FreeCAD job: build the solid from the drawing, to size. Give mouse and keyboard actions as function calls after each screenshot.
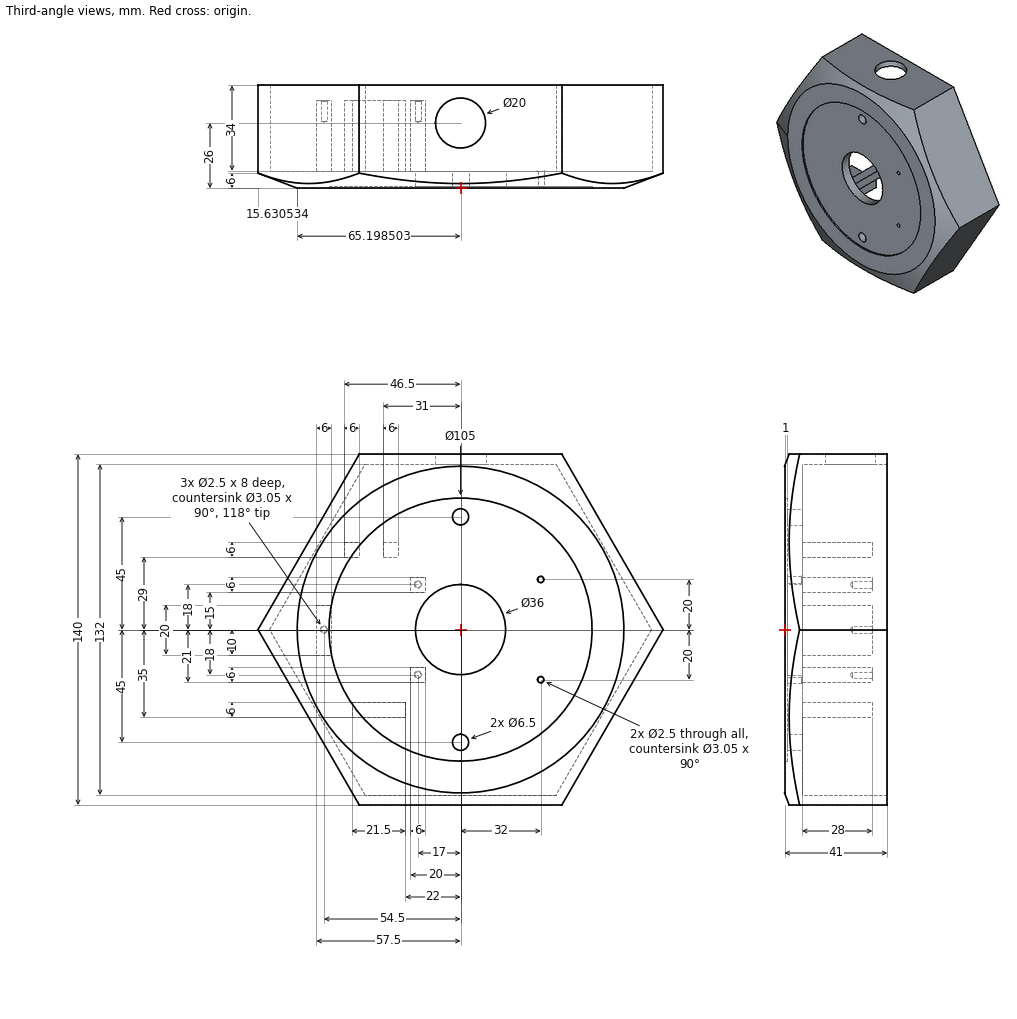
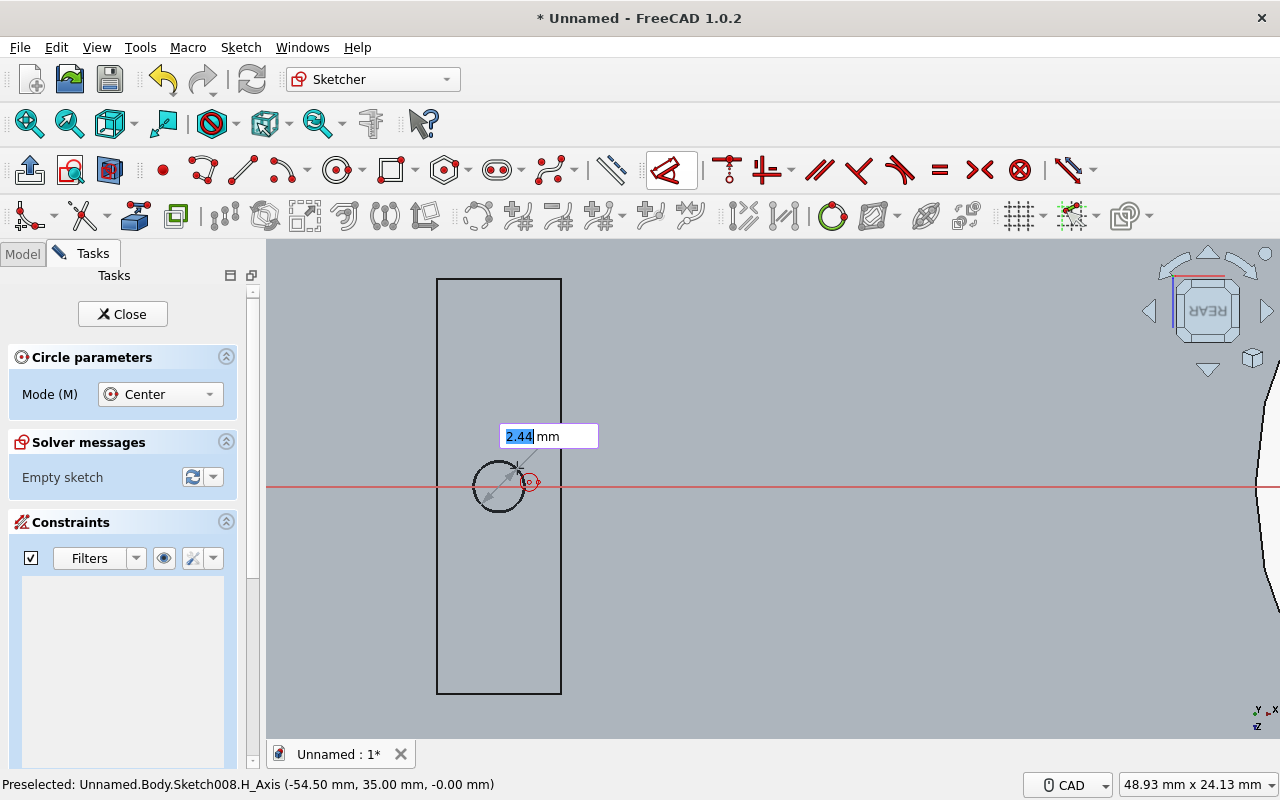
text(2.5)
key(Return)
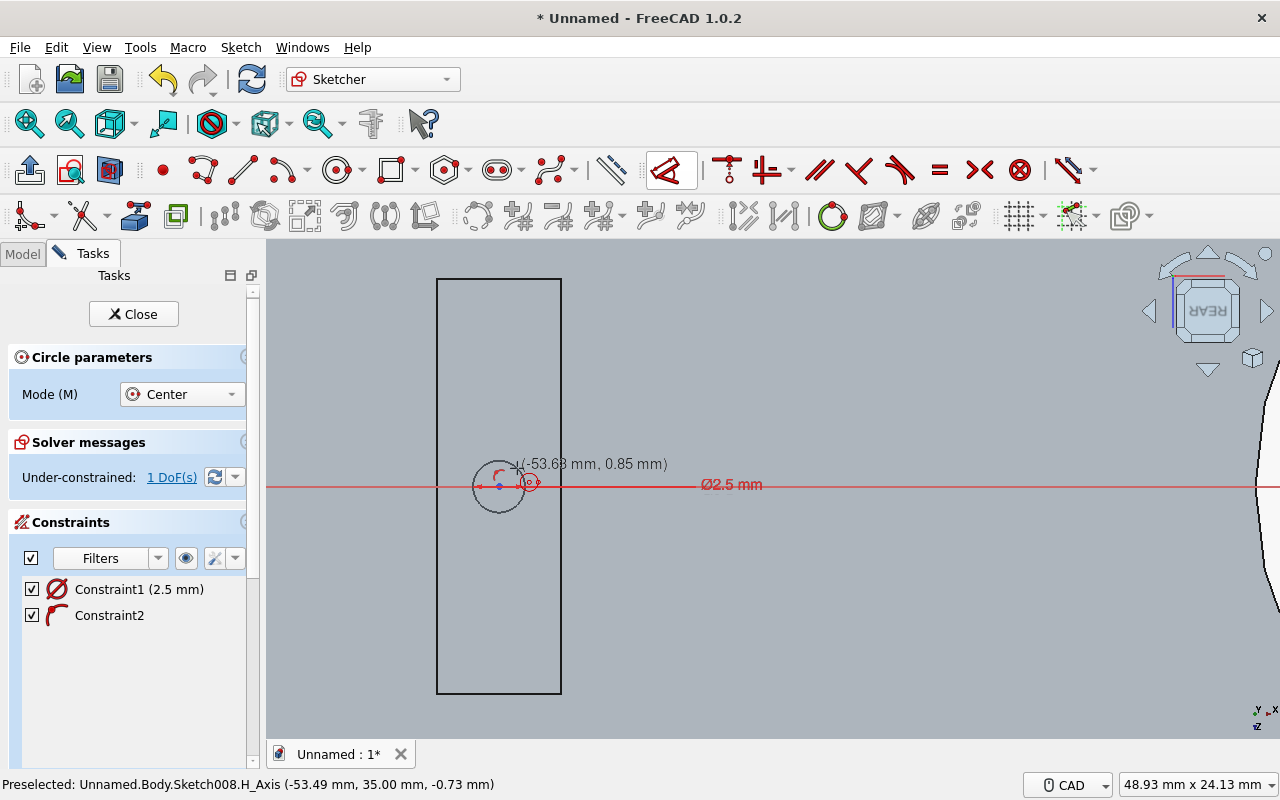
scroll(503, 490, down, 5)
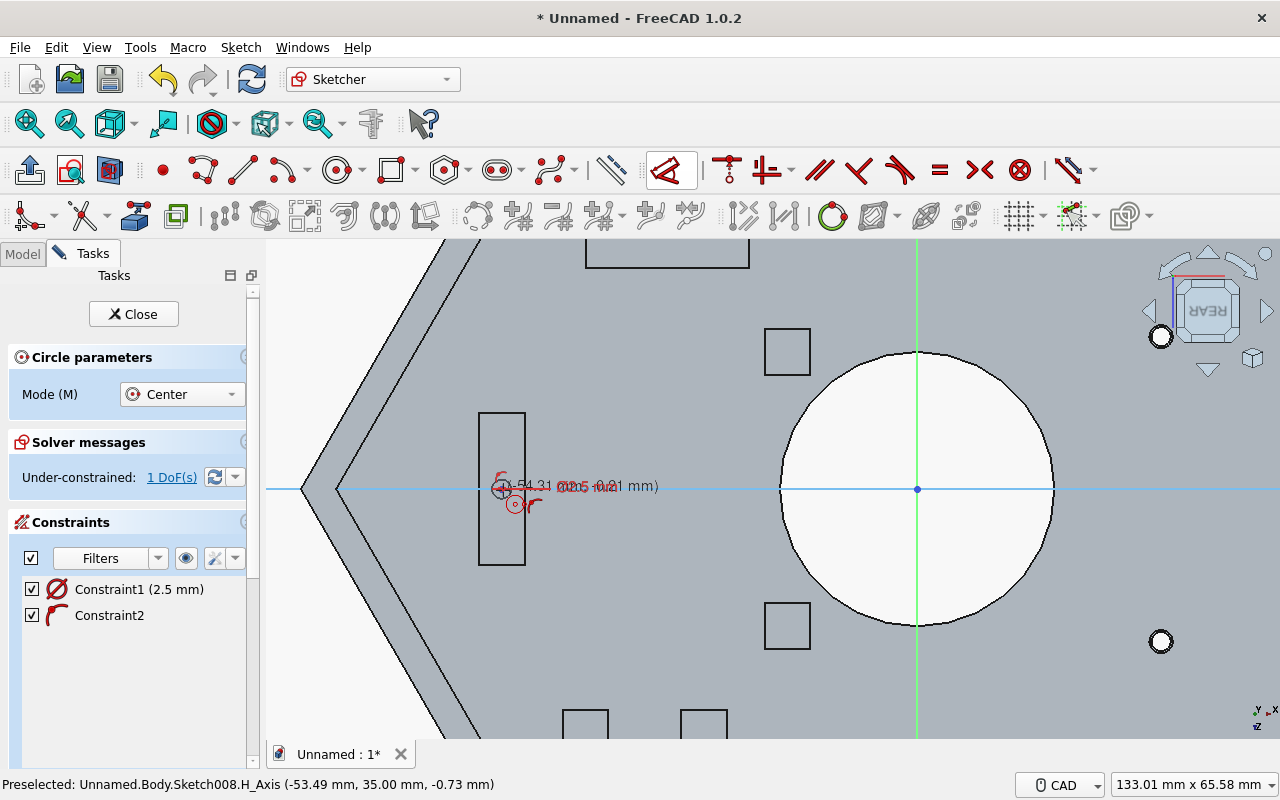
scroll(788, 352, up, 5)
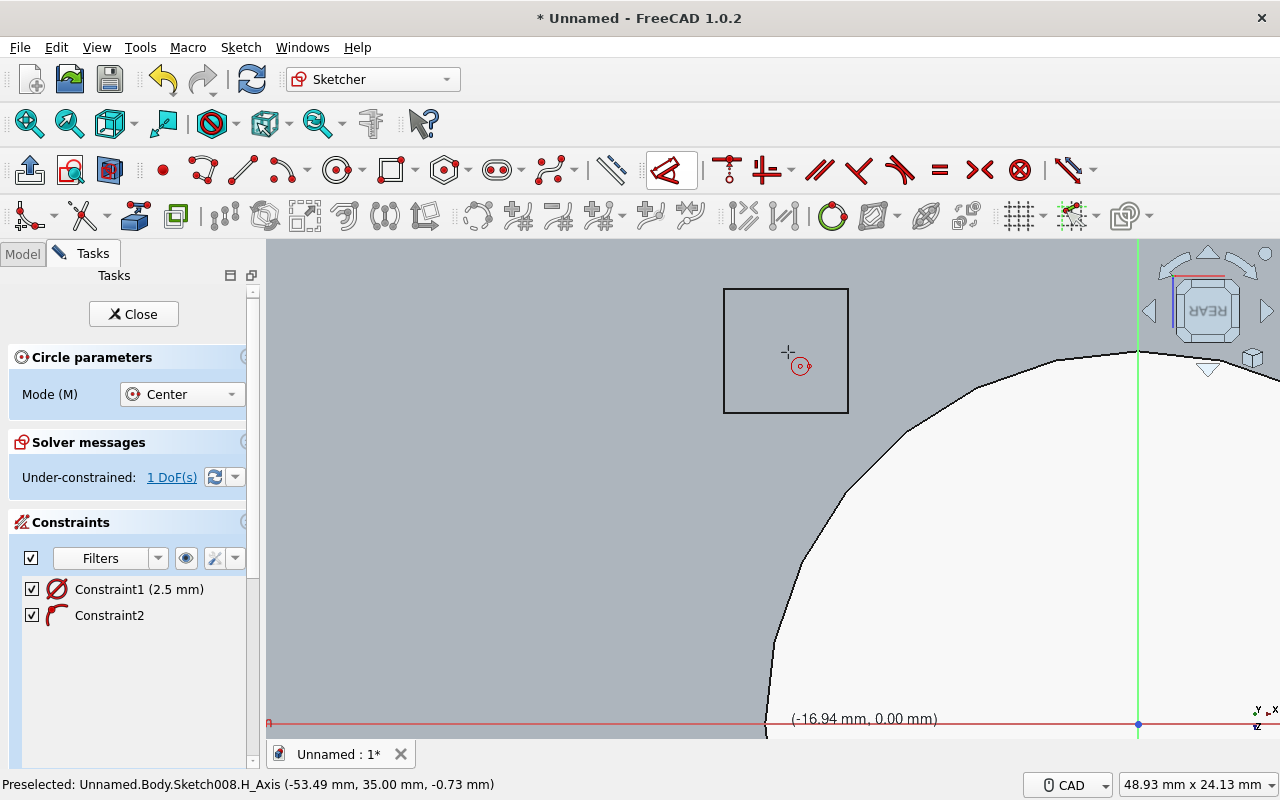
click(786, 351)
move(804, 333)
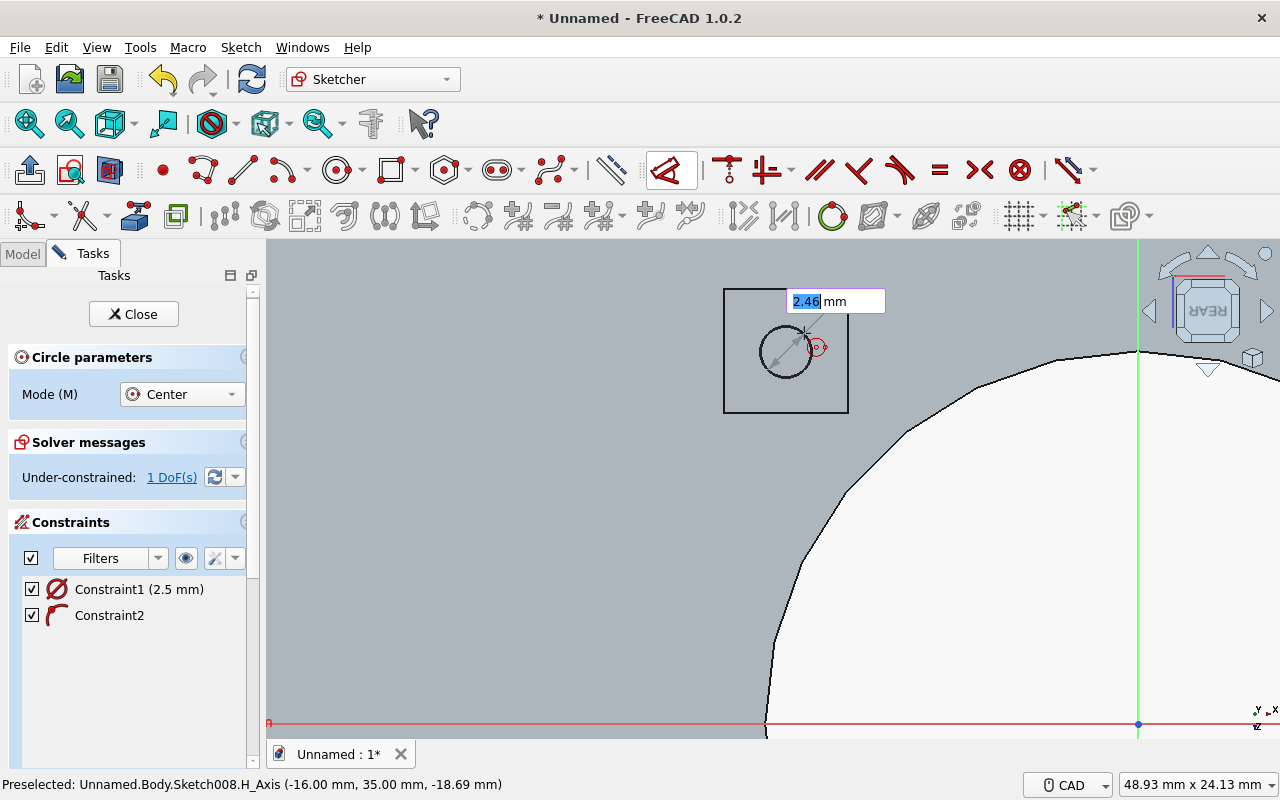
text(2.5)
key(Return)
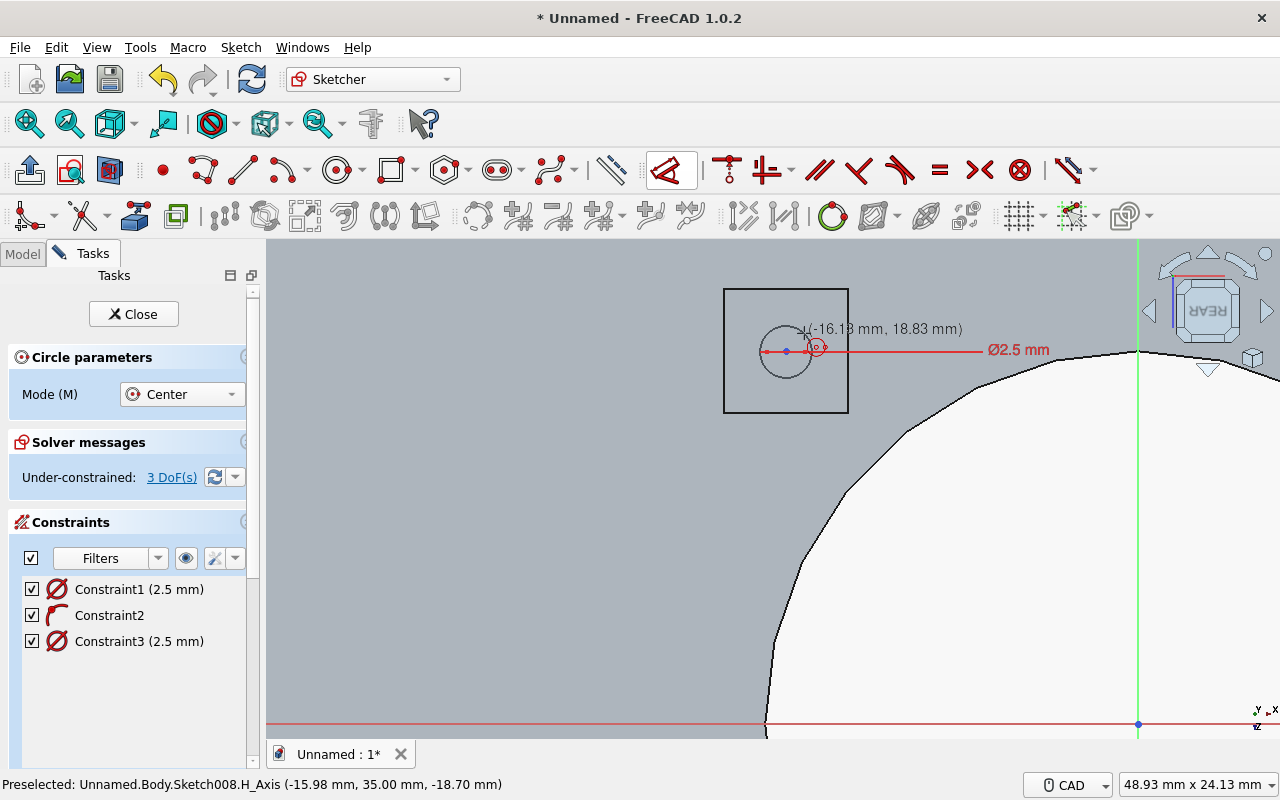
scroll(788, 352, down, 5)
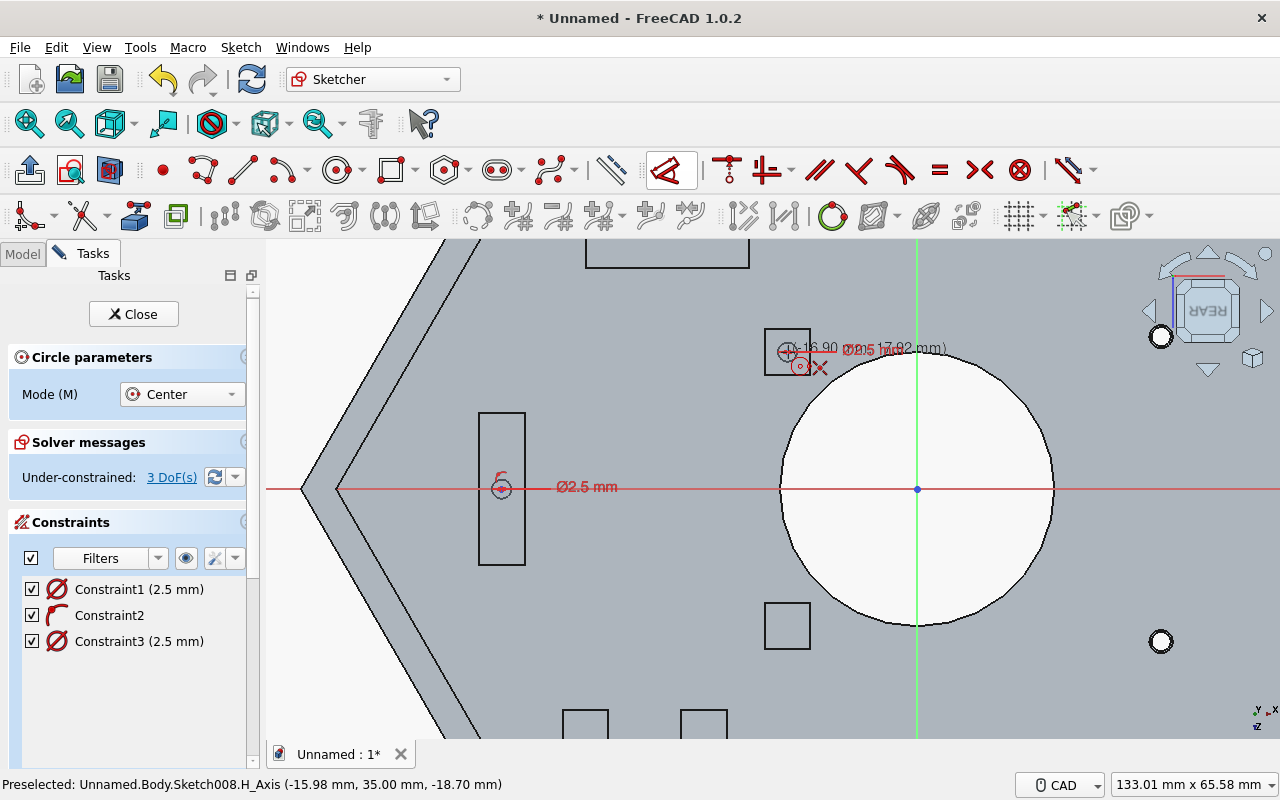
scroll(788, 626, up, 5)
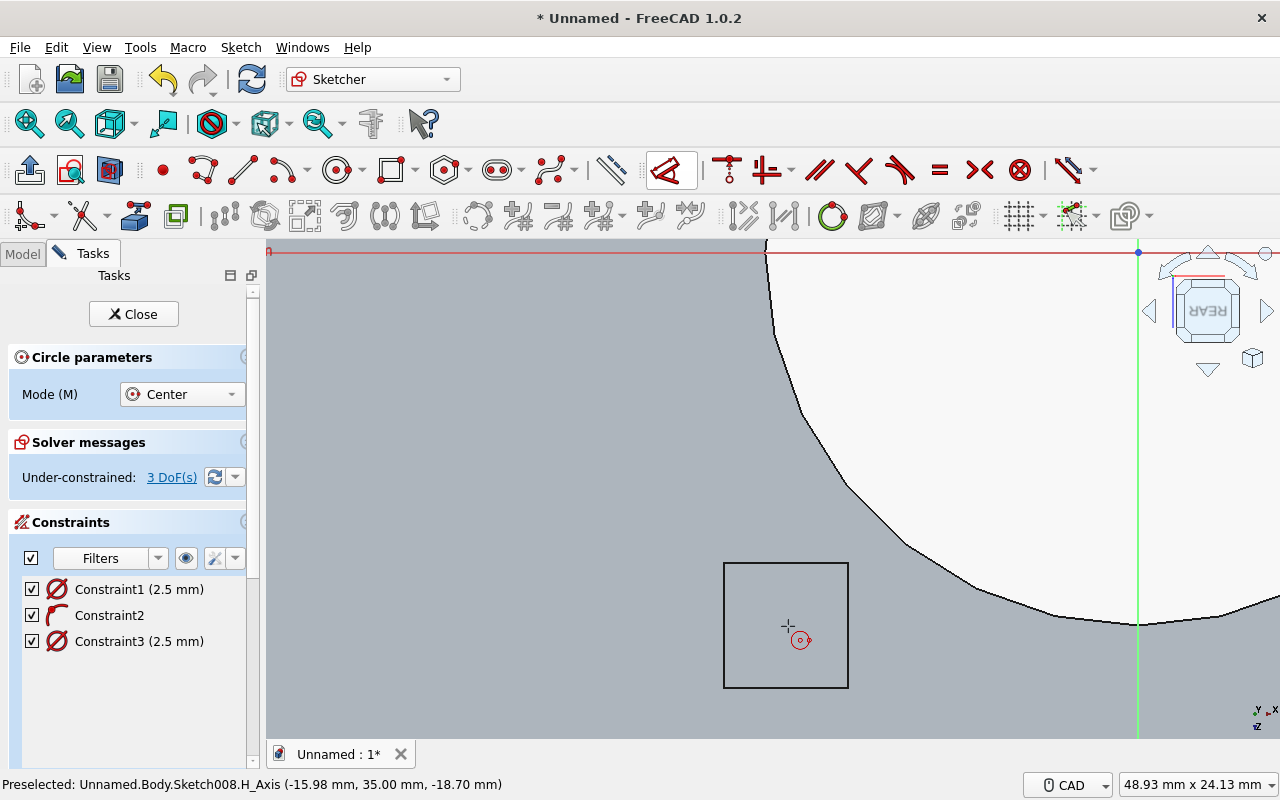
click(786, 626)
move(804, 607)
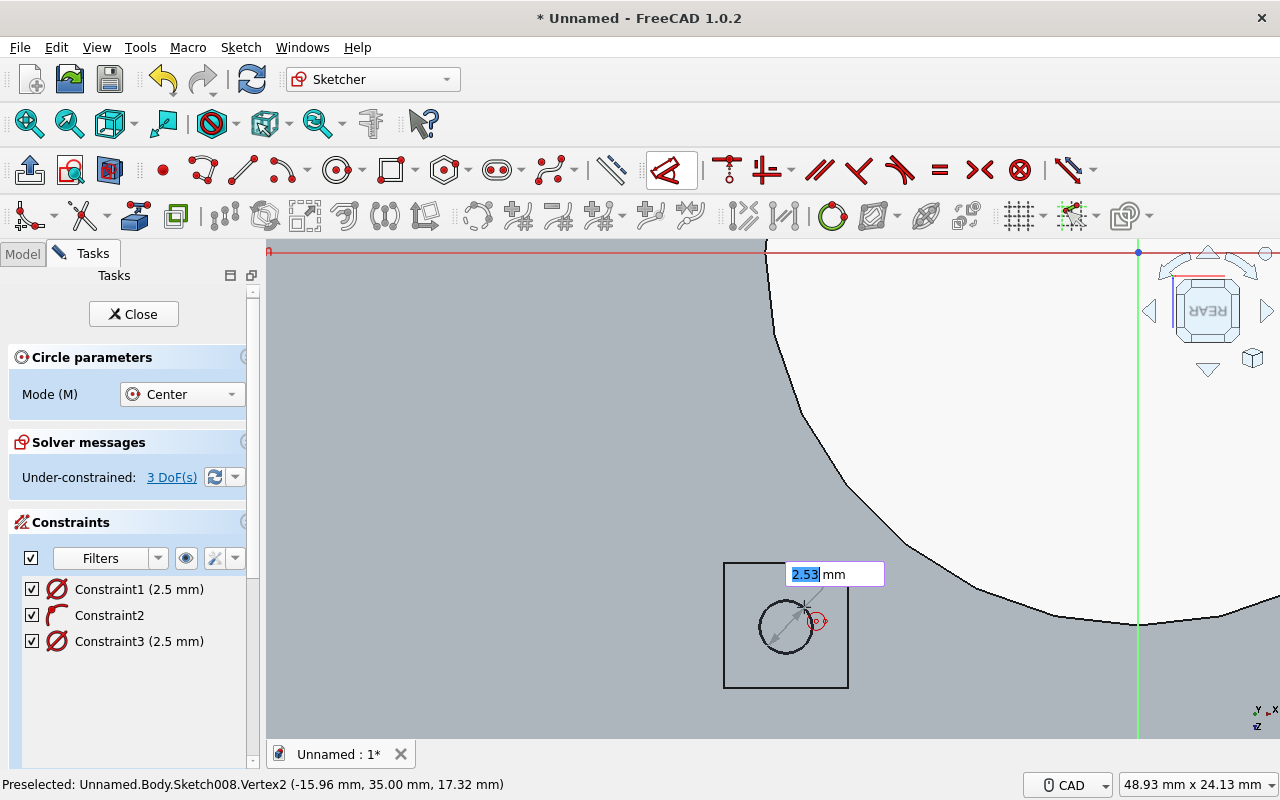
text(2.5)
key(Return)
key(Escape)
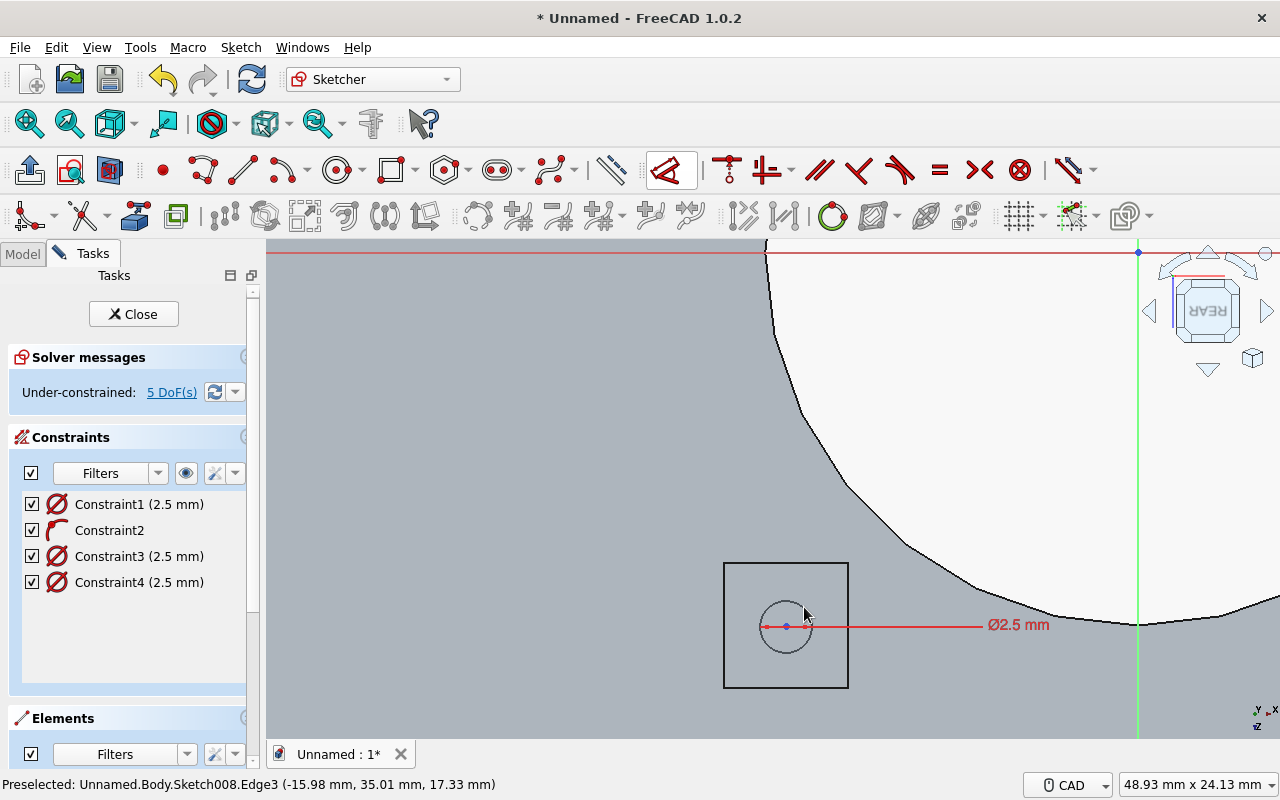
scroll(788, 627, down, 5)